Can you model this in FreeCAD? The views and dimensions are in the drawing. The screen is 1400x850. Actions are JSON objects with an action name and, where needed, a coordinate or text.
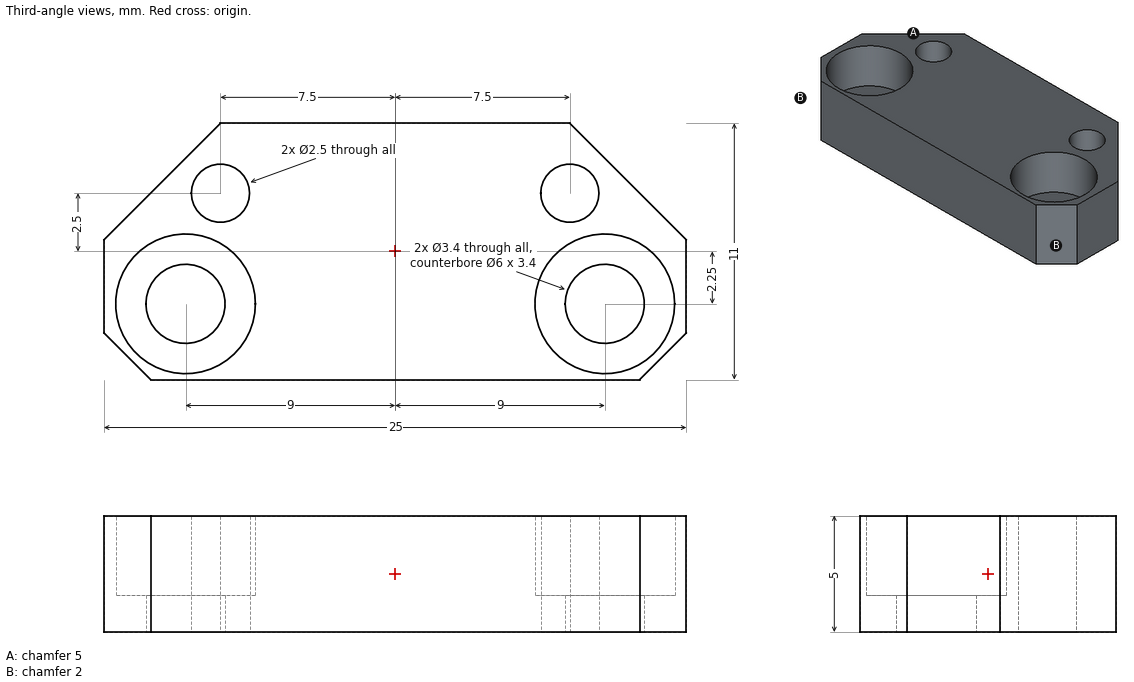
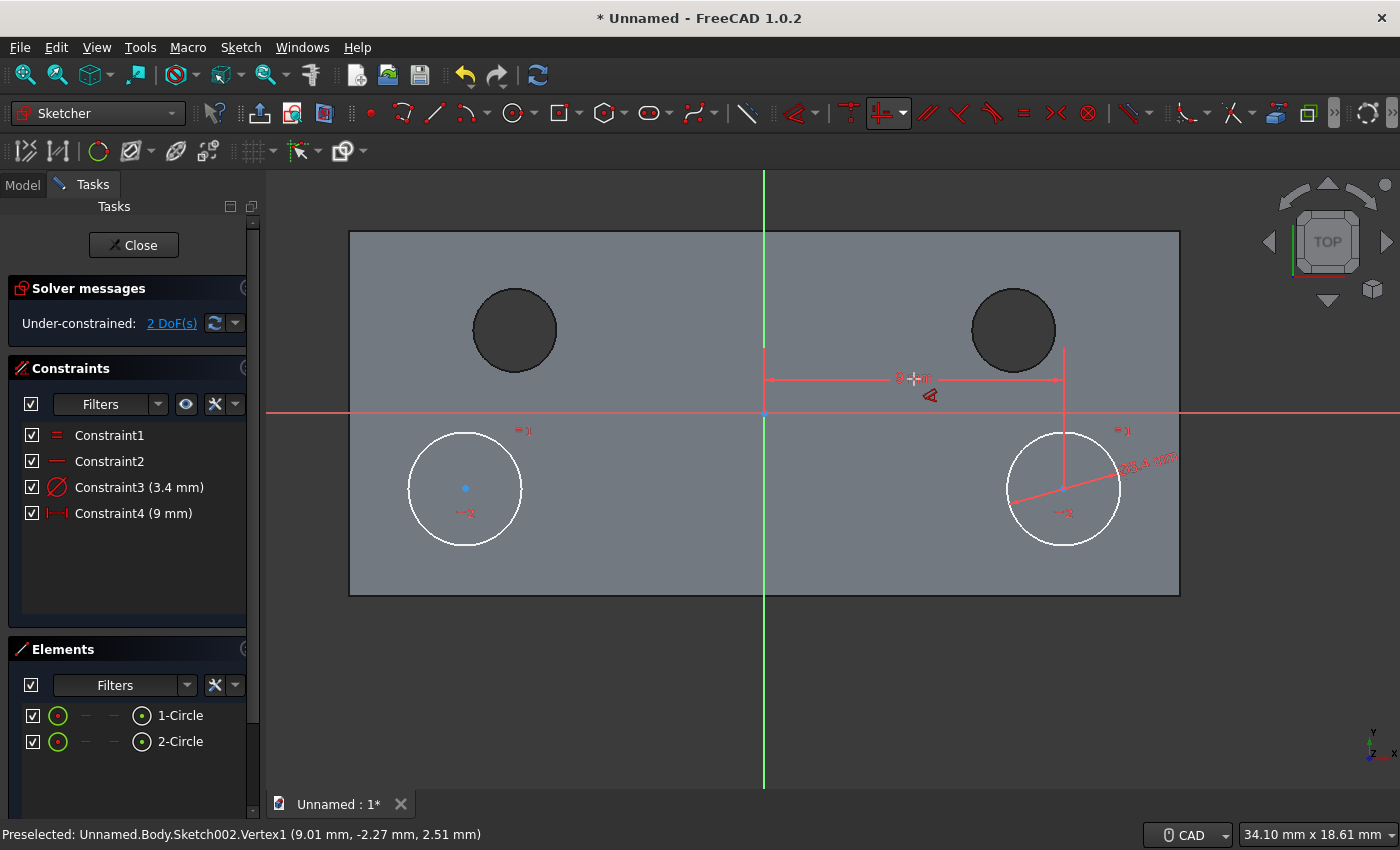
{"action": "left_click", "coordinate": [465, 489]}
{"action": "left_click", "coordinate": [615, 379]}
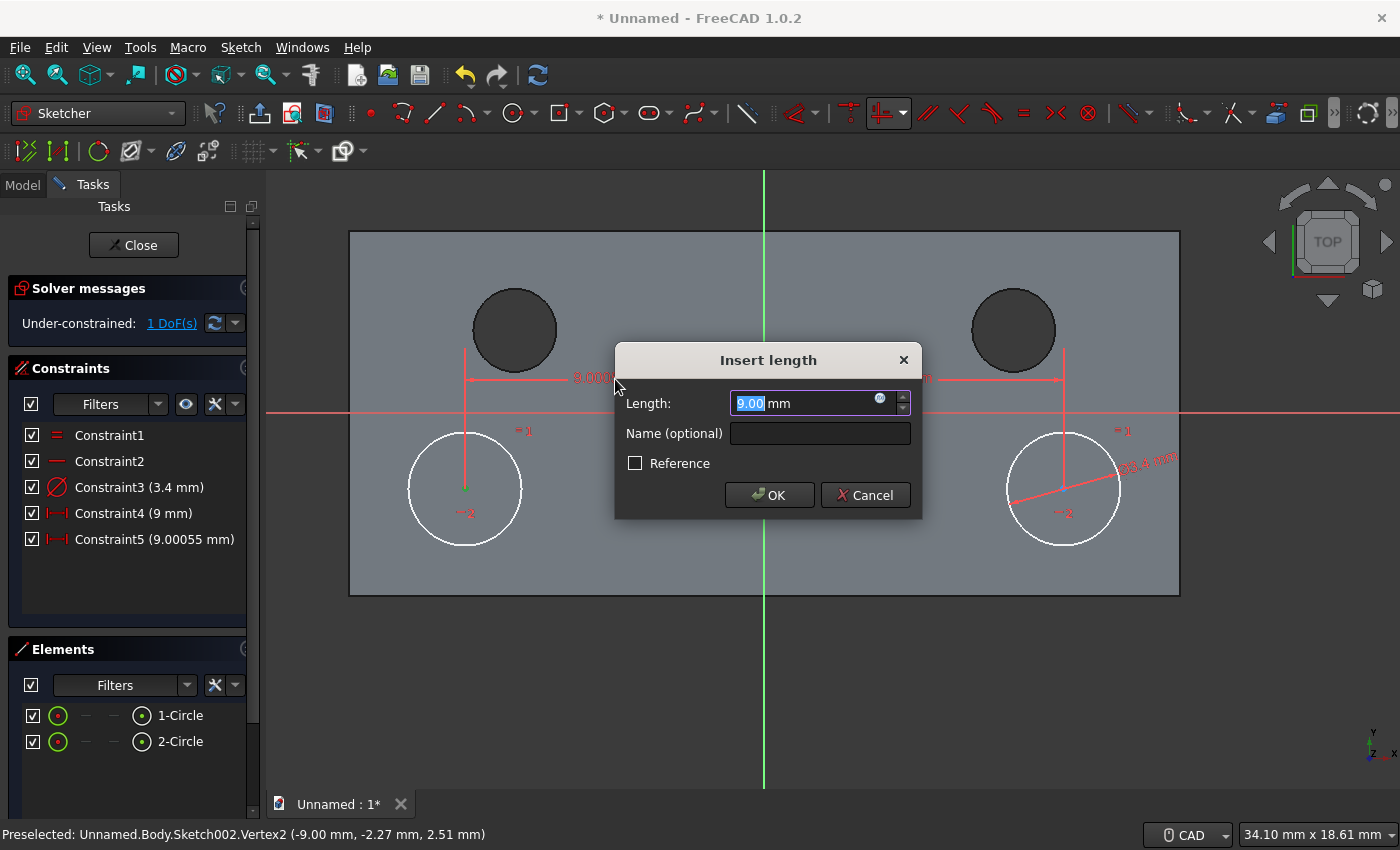
{"action": "type", "text": "9"}
{"action": "key", "text": "Return"}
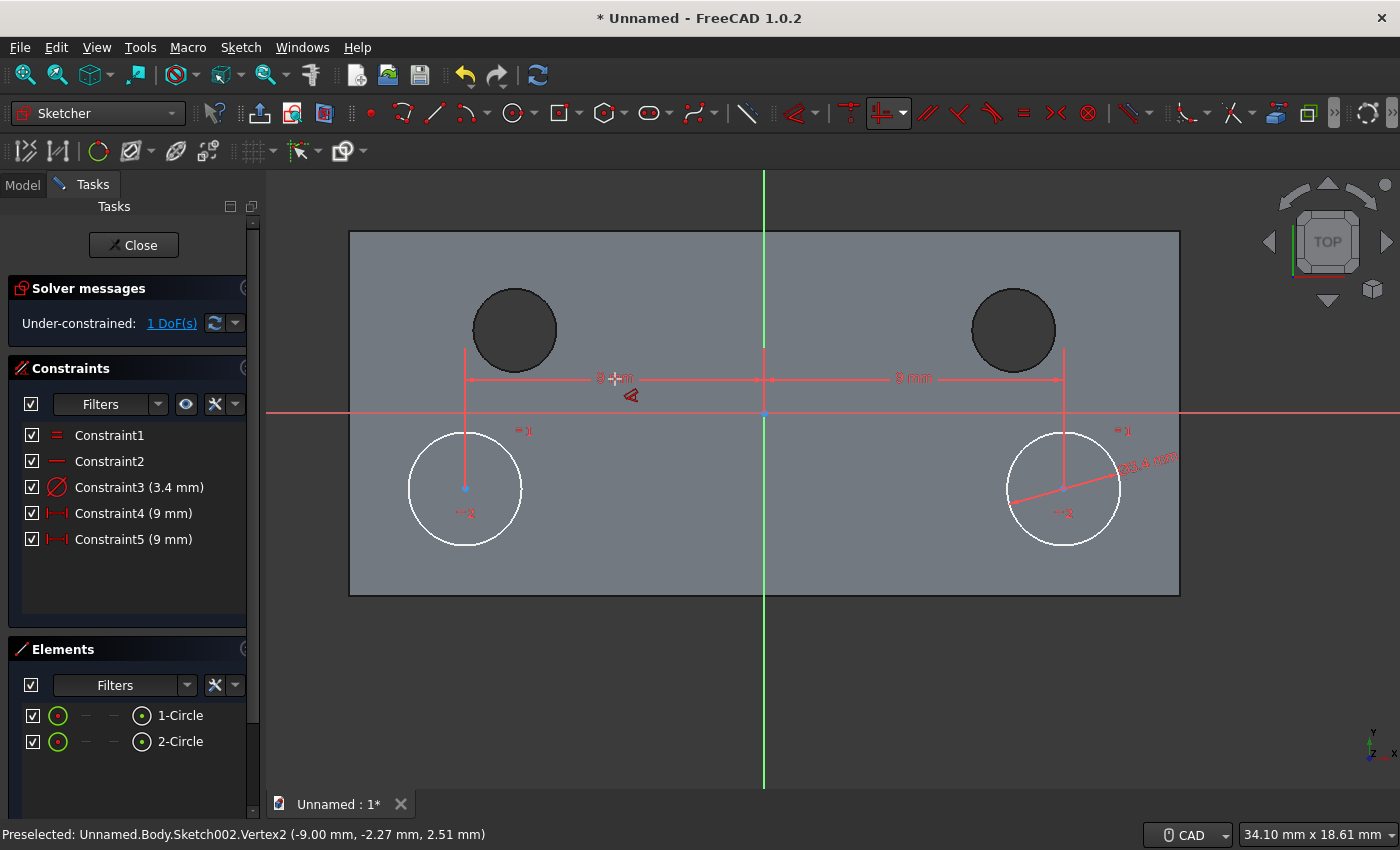
{"action": "left_click", "coordinate": [1064, 489]}
{"action": "left_click", "coordinate": [730, 451]}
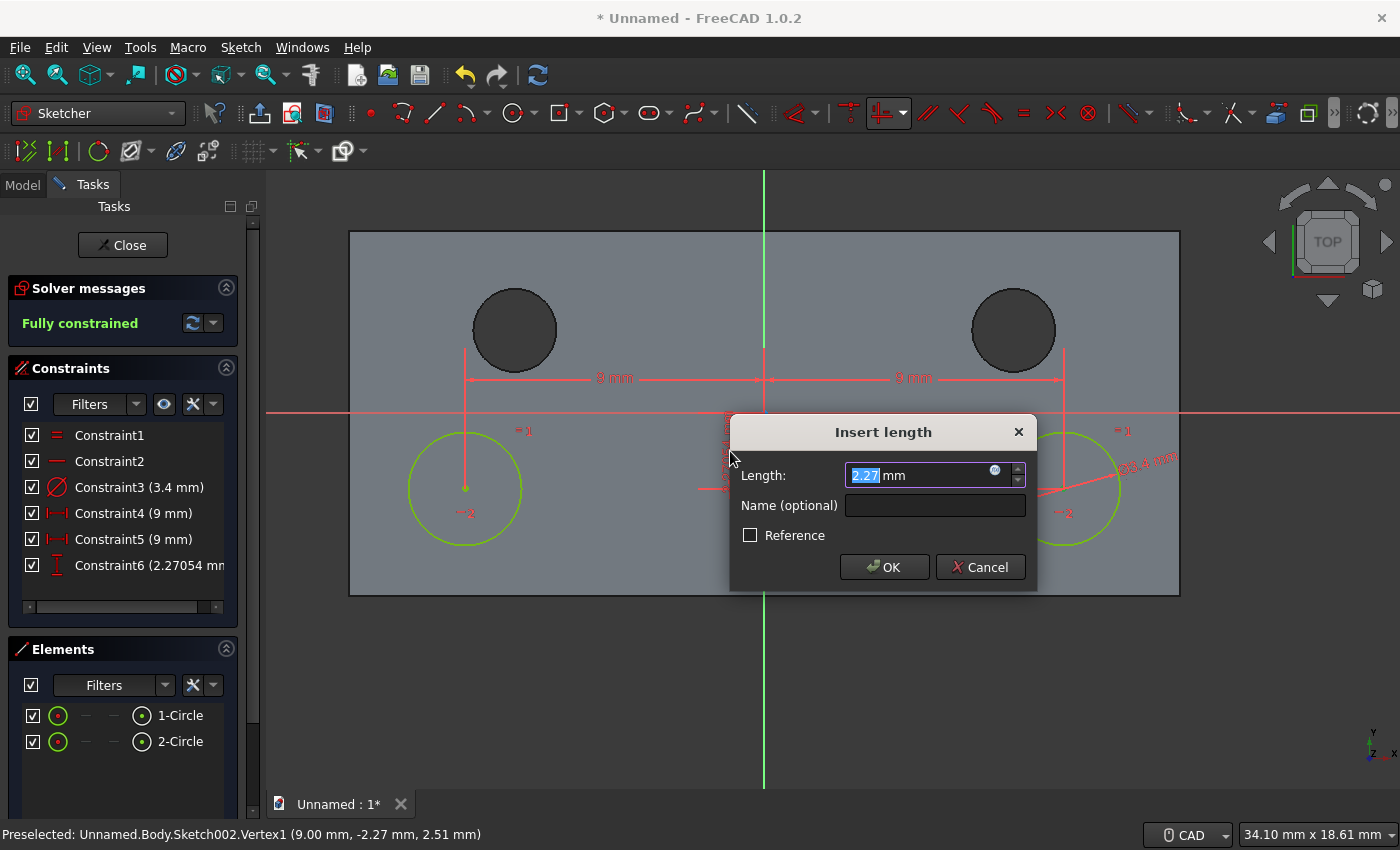
{"action": "type", "text": "2.25"}
{"action": "key", "text": "Return"}
{"action": "key", "text": "Escape"}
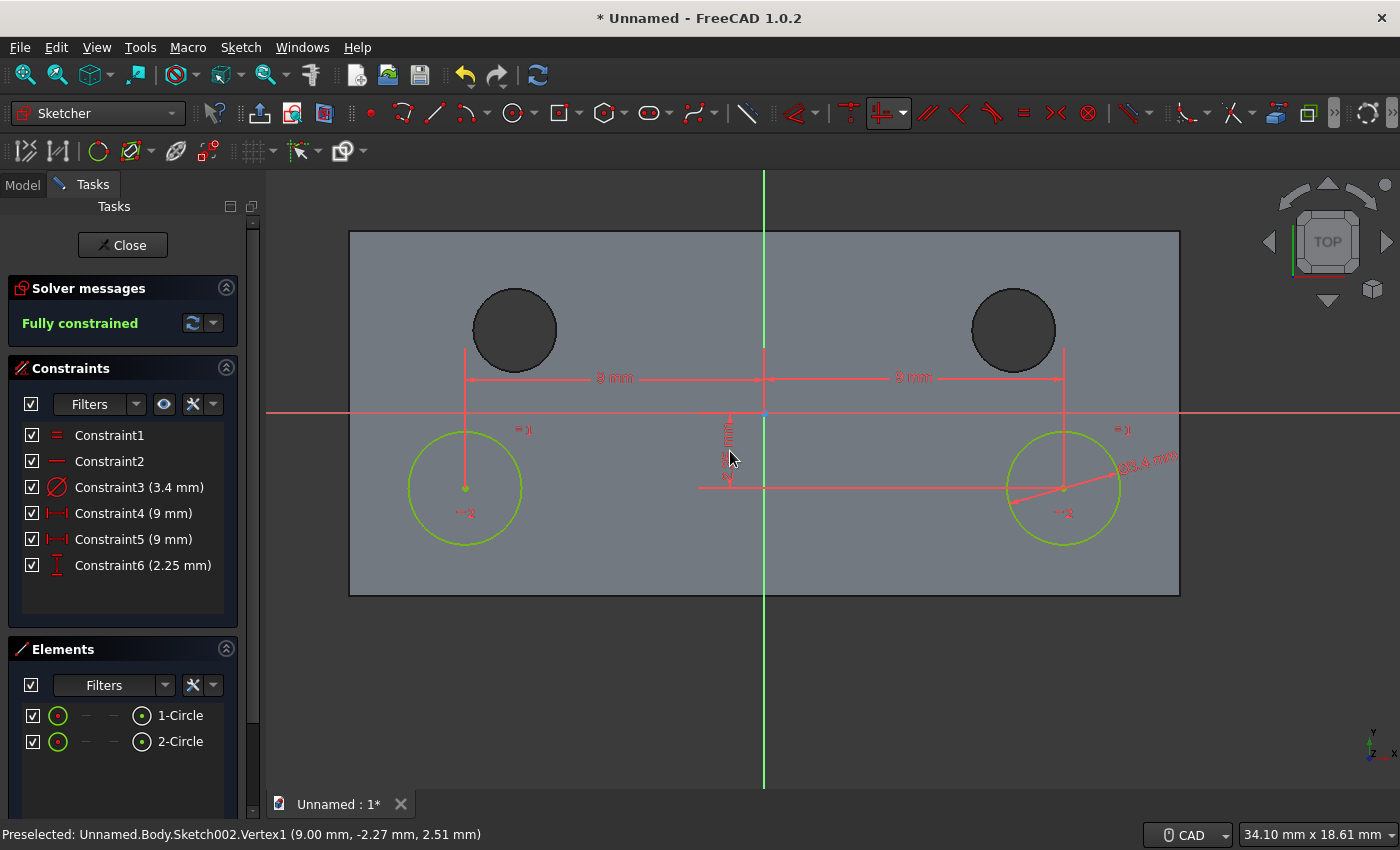
{"action": "left_click", "coordinate": [123, 245]}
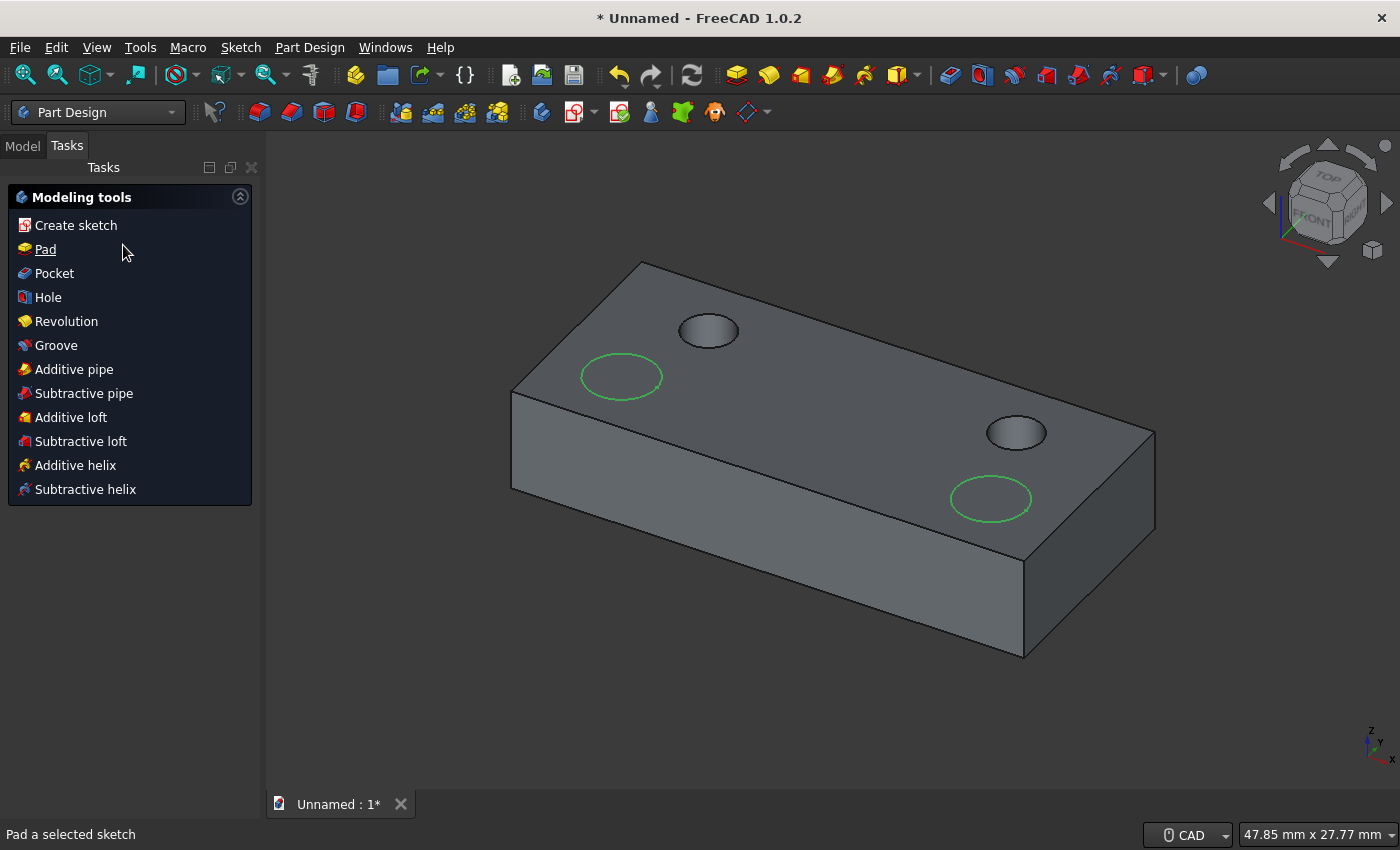
{"action": "left_click", "coordinate": [984, 76]}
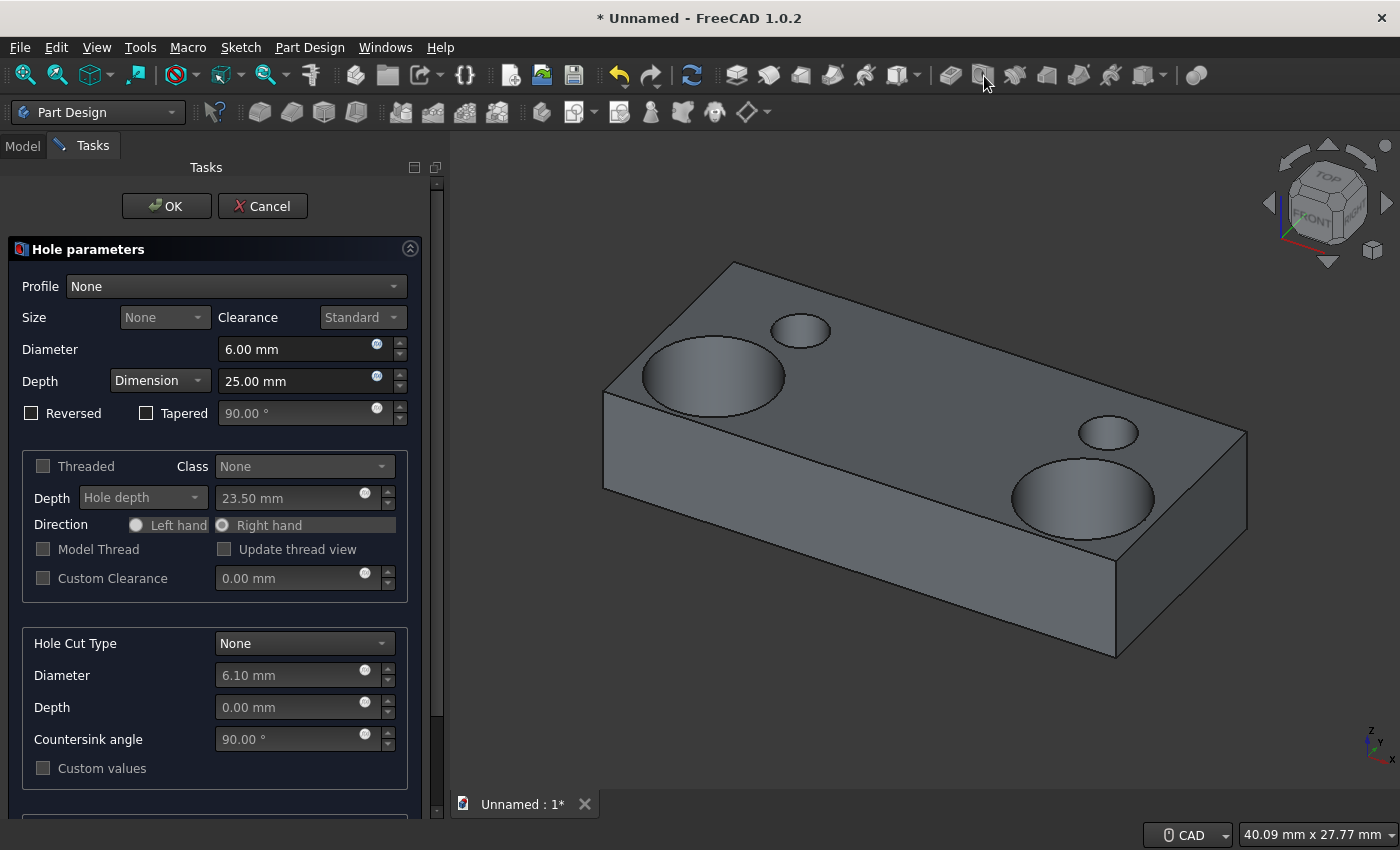
{"action": "triple_click", "coordinate": [305, 349]}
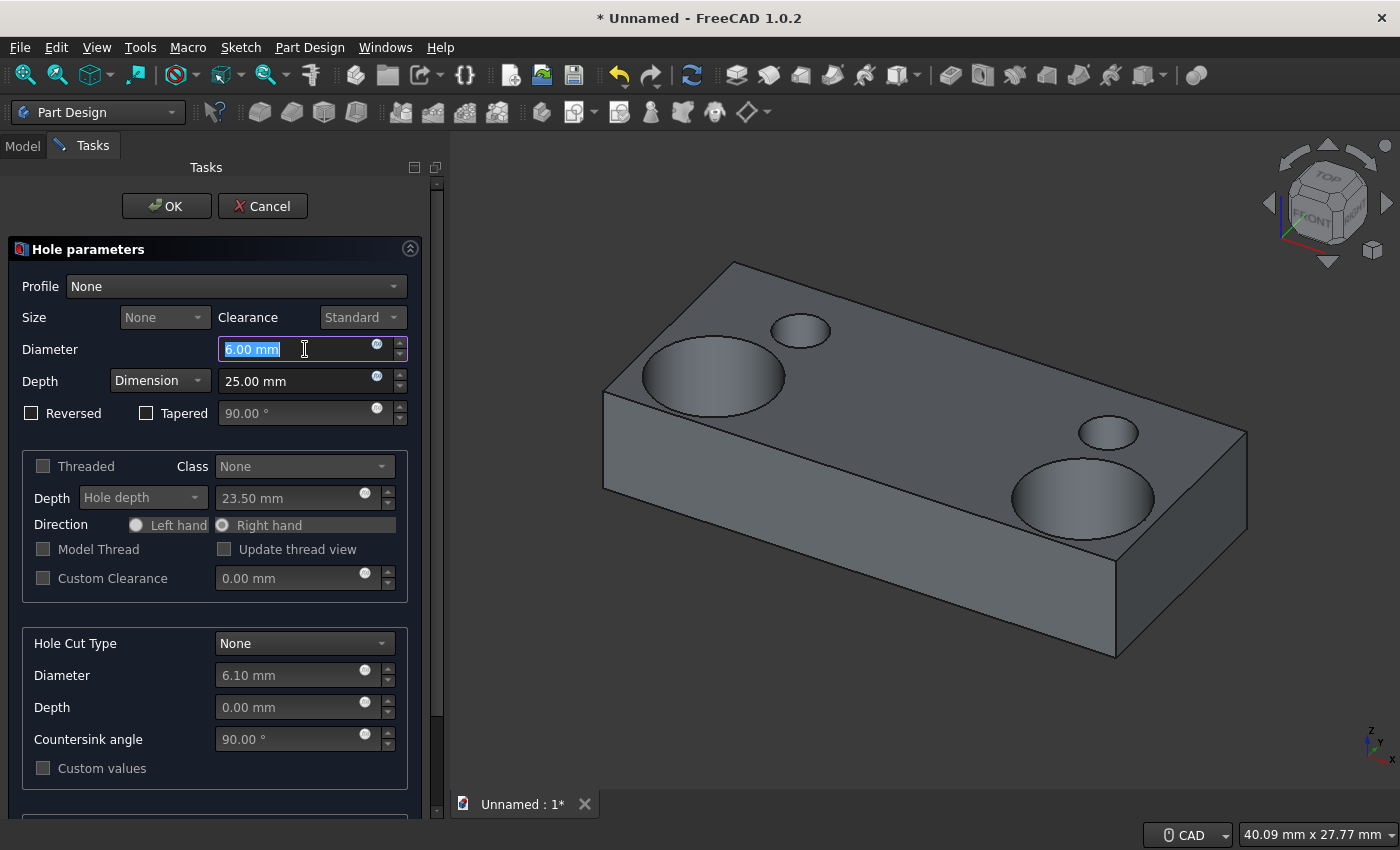
{"action": "type", "text": "3.4"}
{"action": "key", "text": "Tab"}